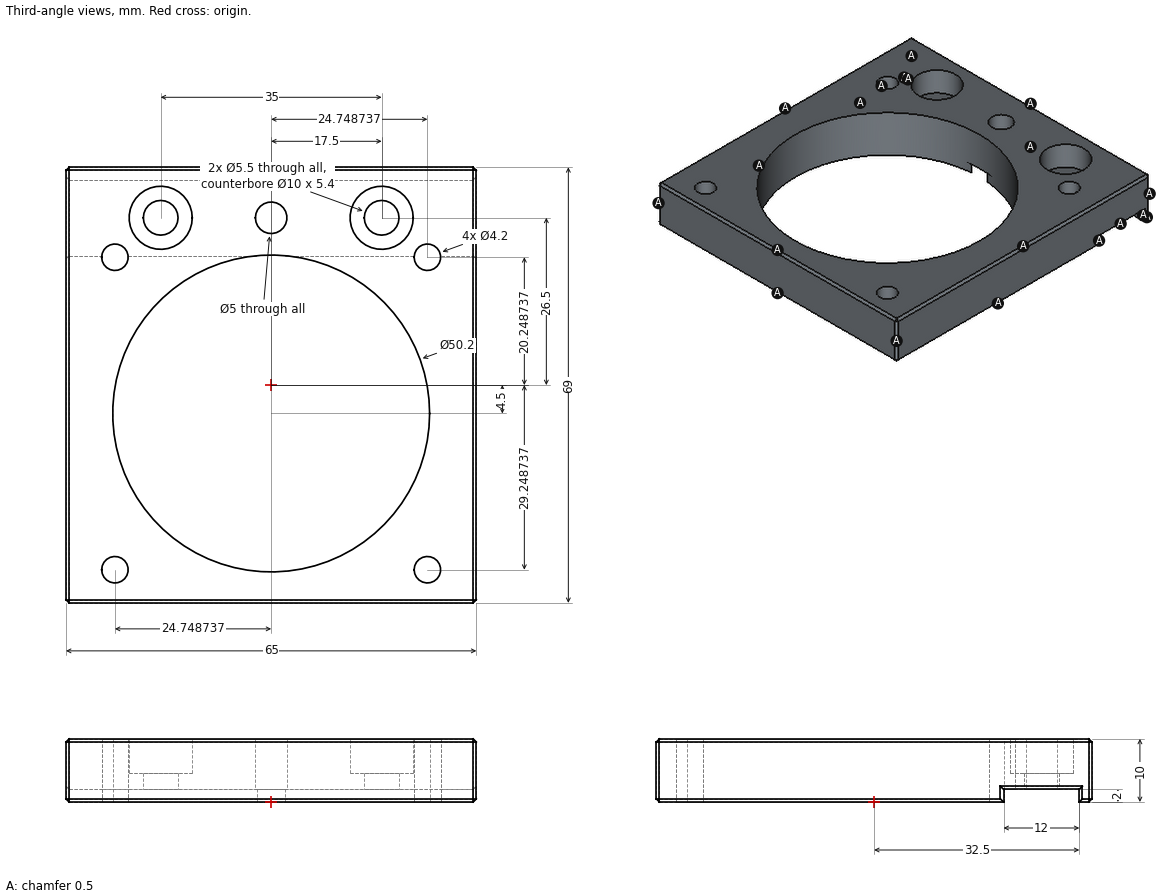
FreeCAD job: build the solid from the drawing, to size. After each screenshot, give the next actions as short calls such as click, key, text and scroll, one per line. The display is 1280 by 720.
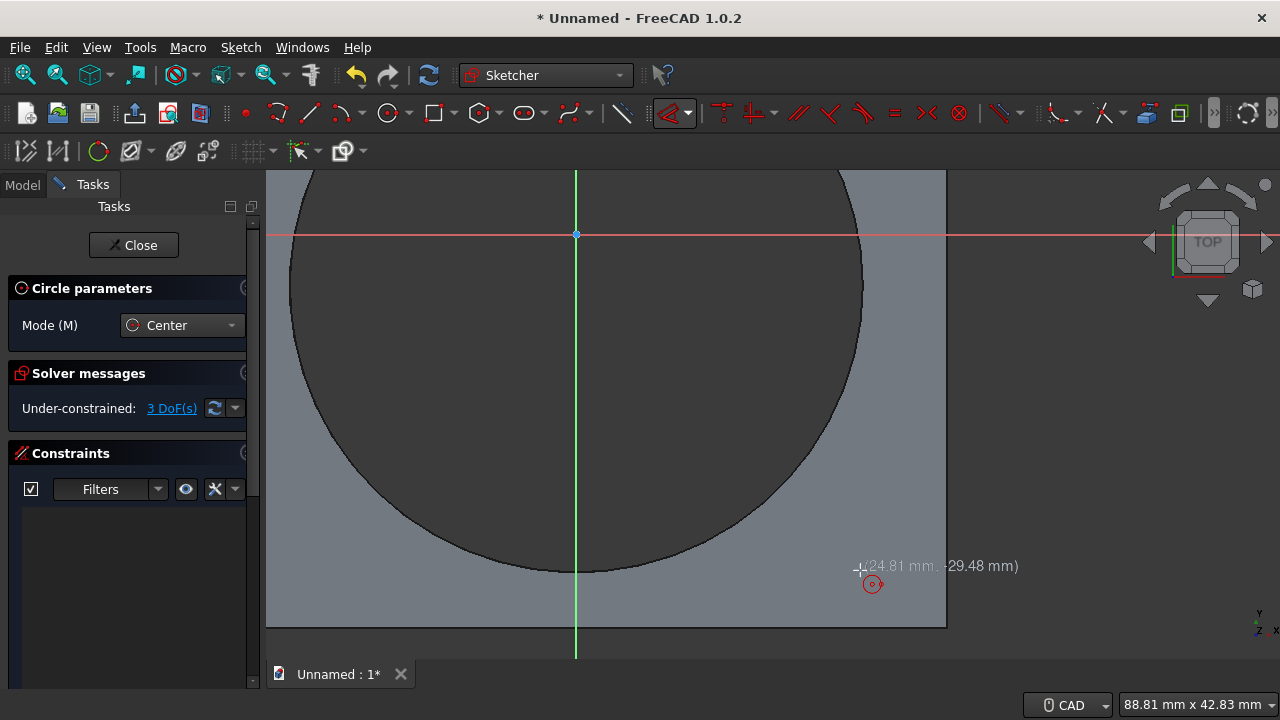
click(859, 568)
click(876, 552)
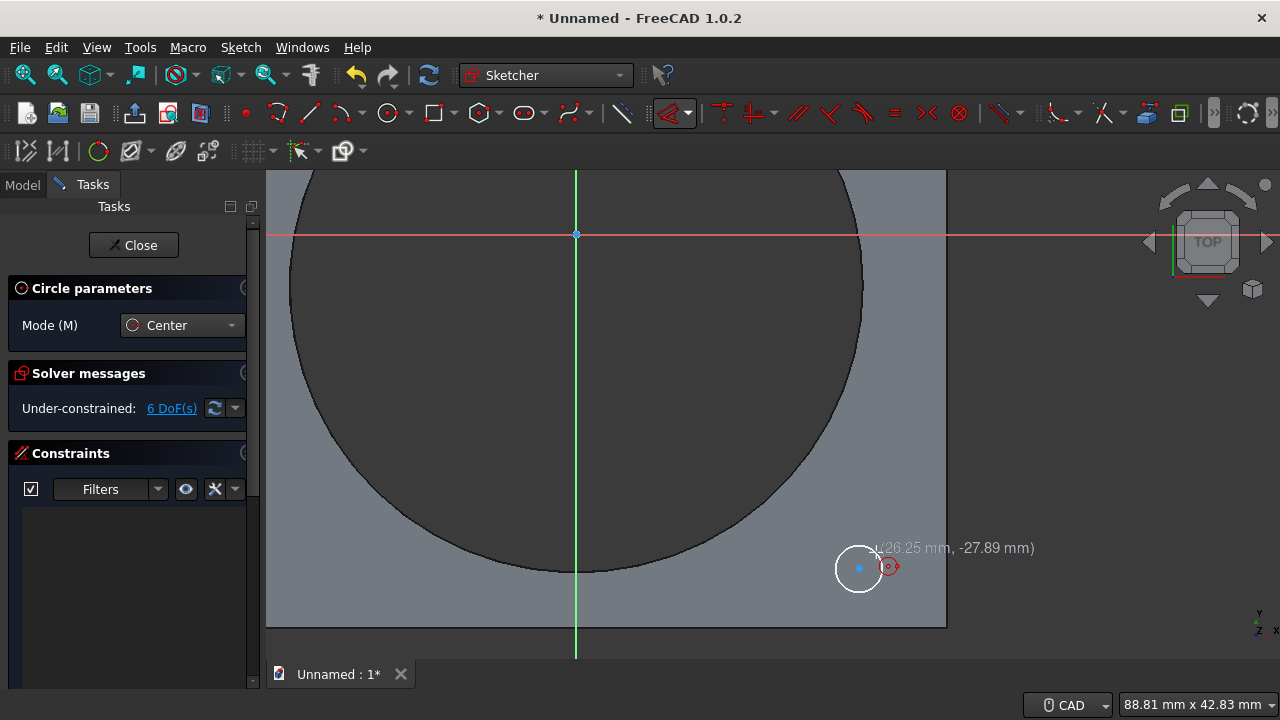
scroll(860, 571, down, 3)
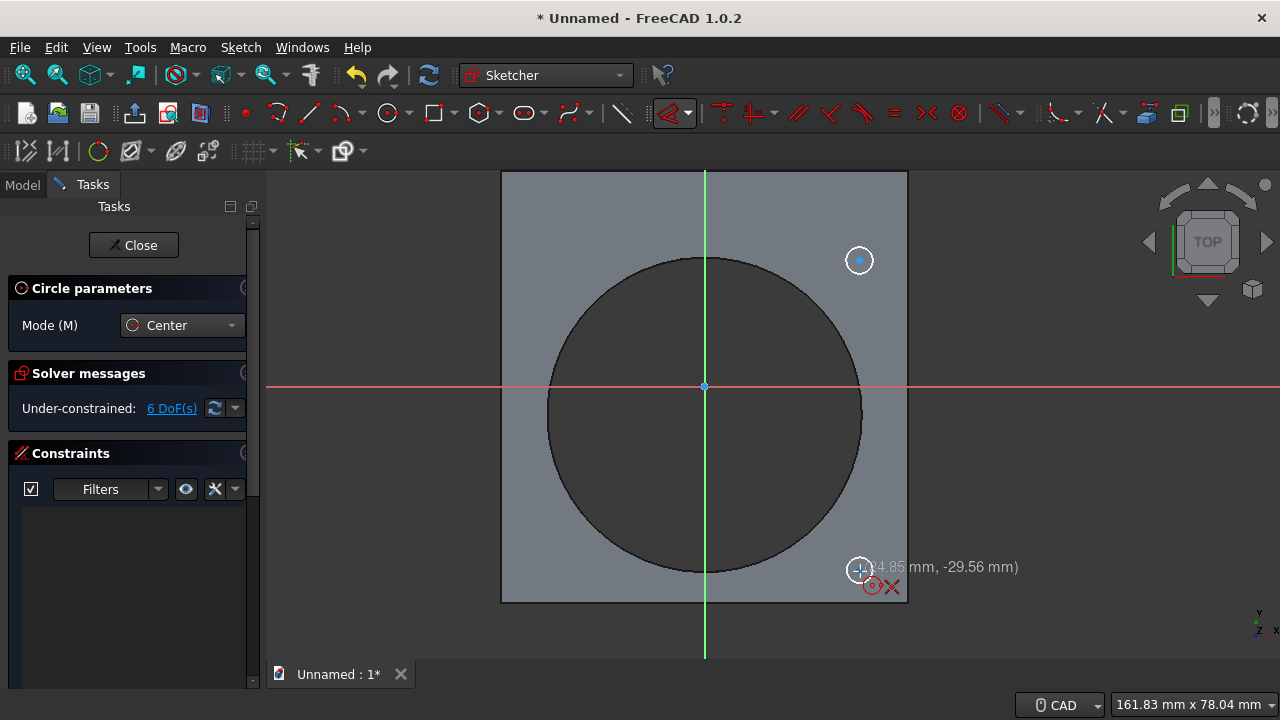
scroll(549, 570, up, 3)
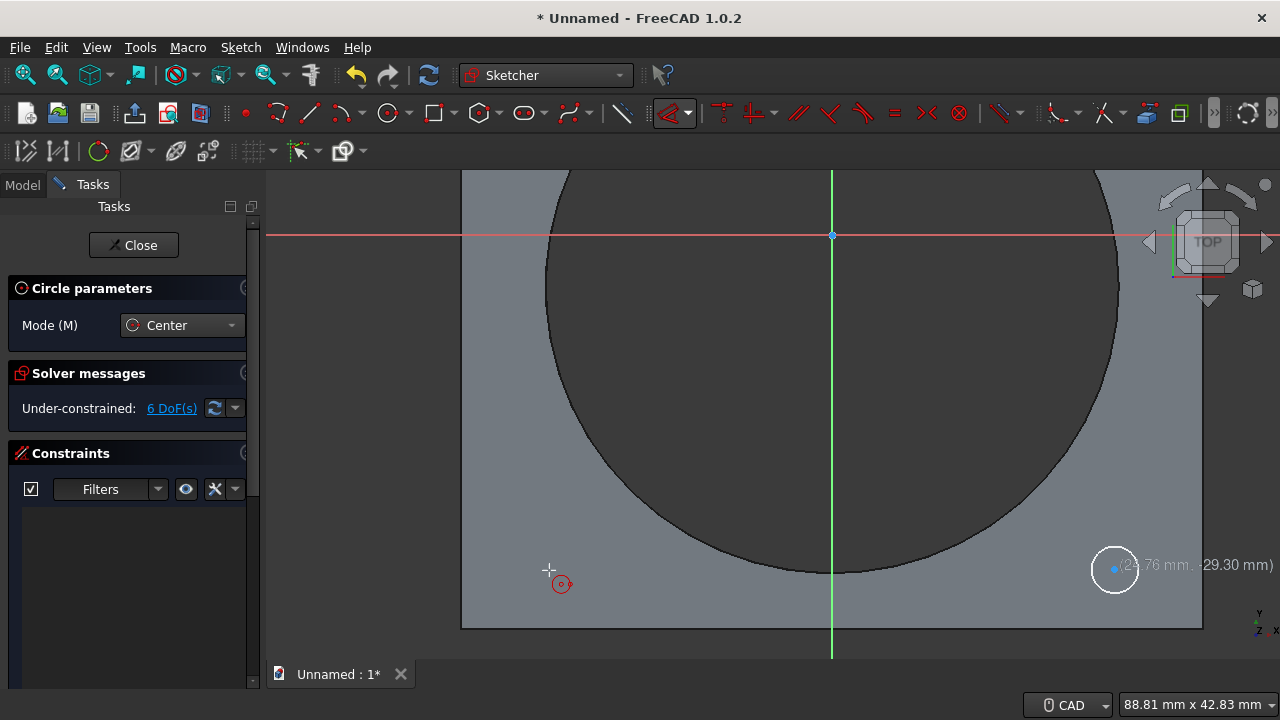
click(550, 569)
click(567, 552)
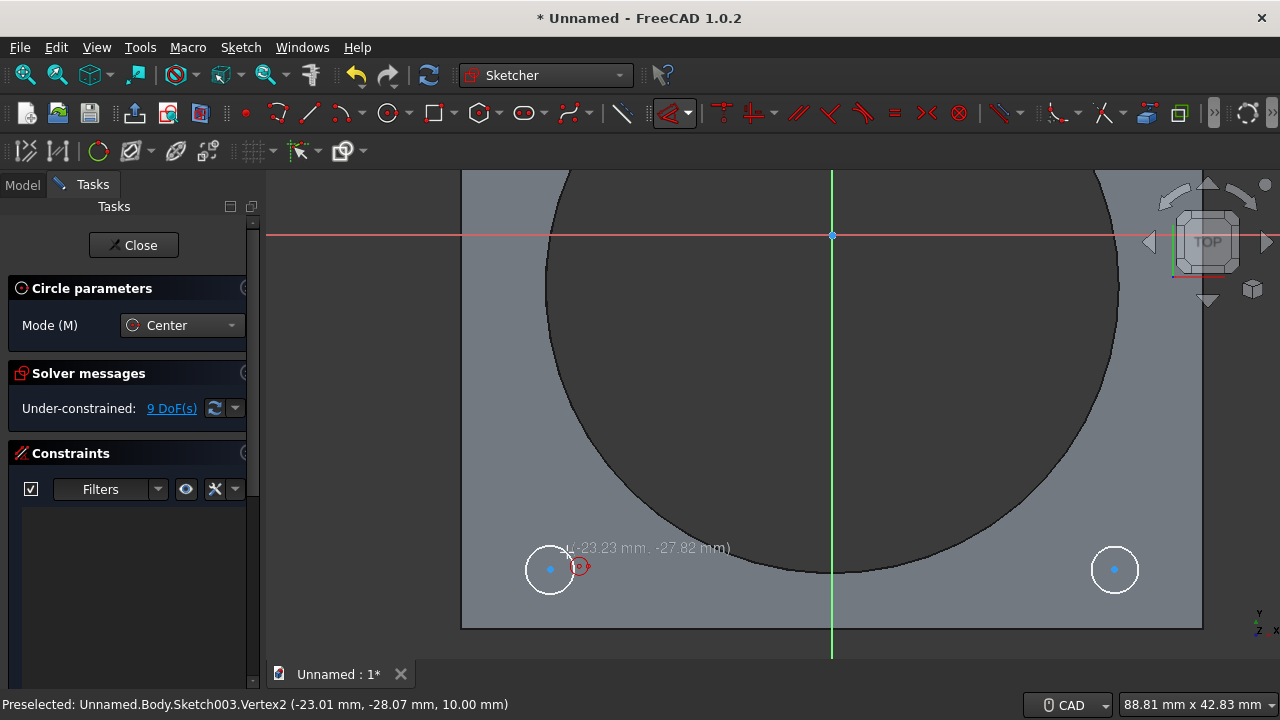
scroll(549, 570, down, 3)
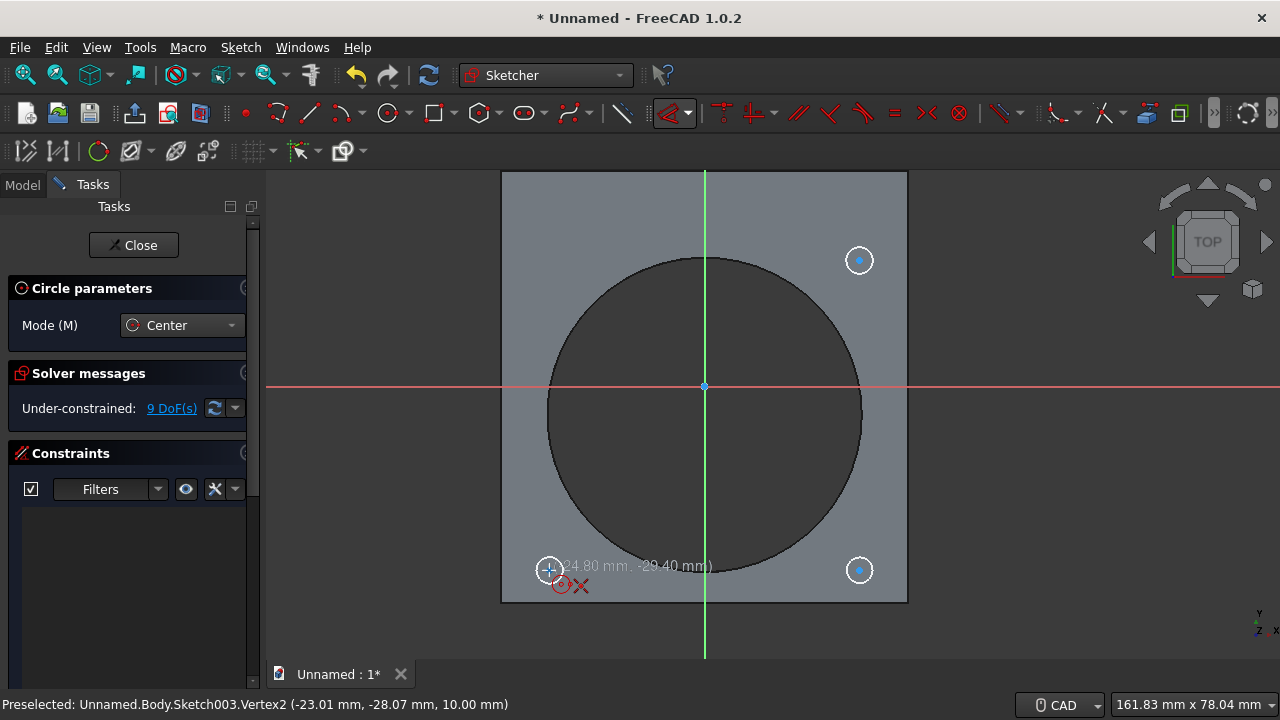
scroll(549, 260, up, 3)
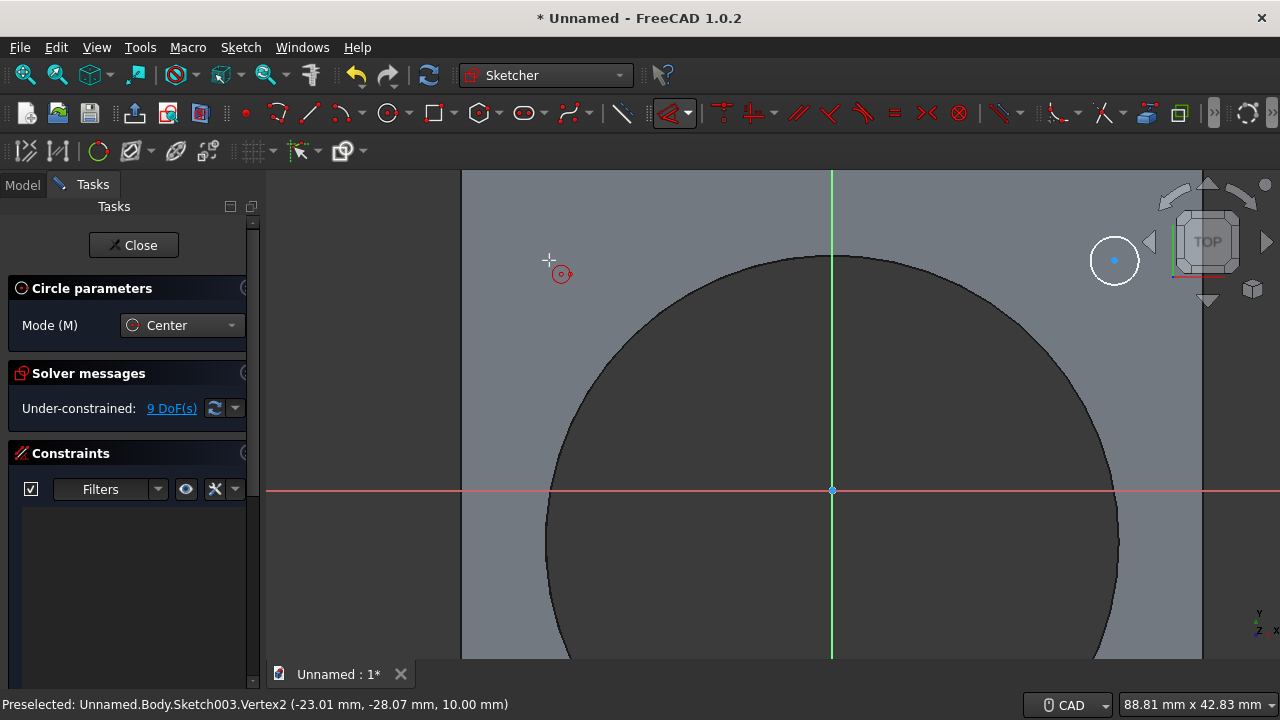
click(550, 260)
click(567, 243)
key(Escape)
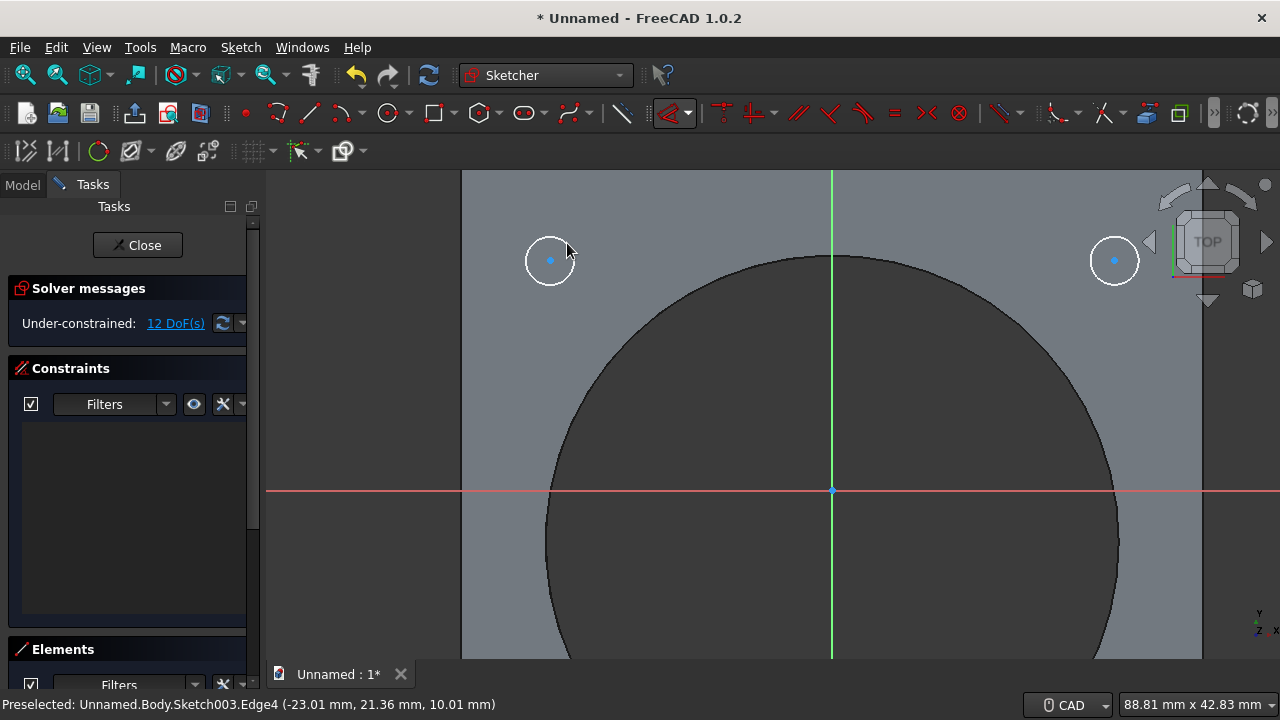
click(1098, 244)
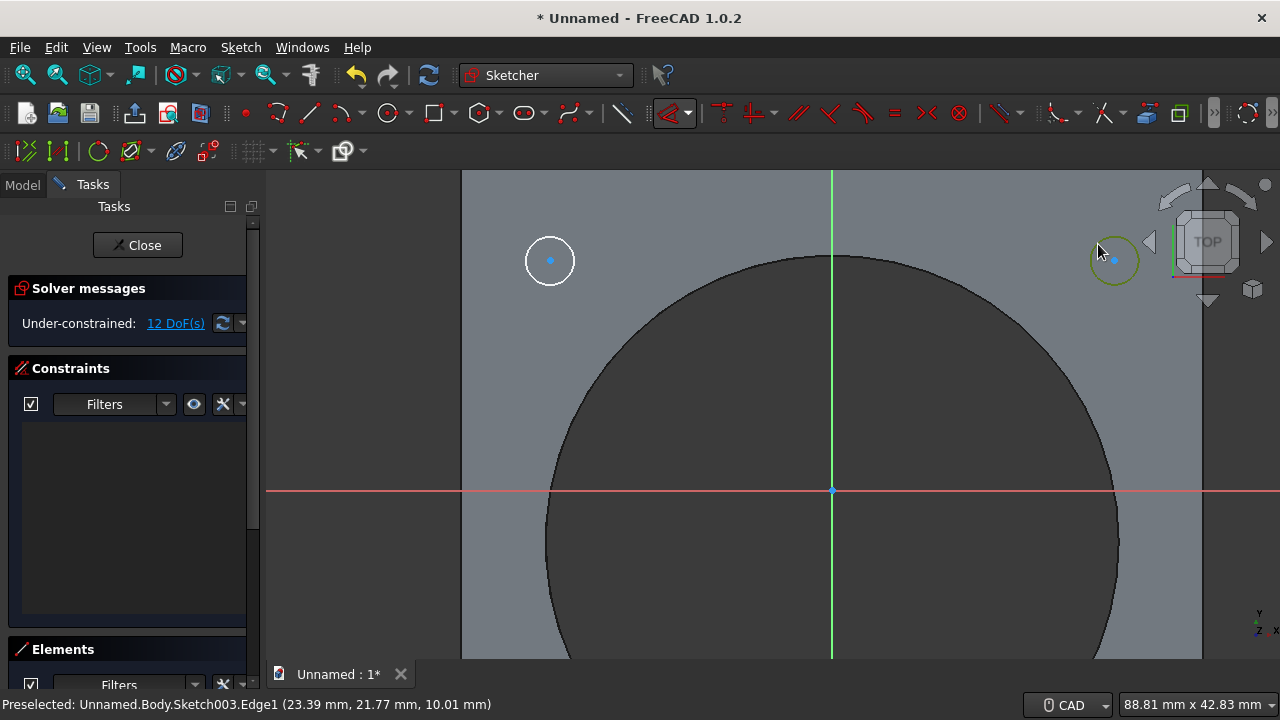
scroll(549, 259, down, 3)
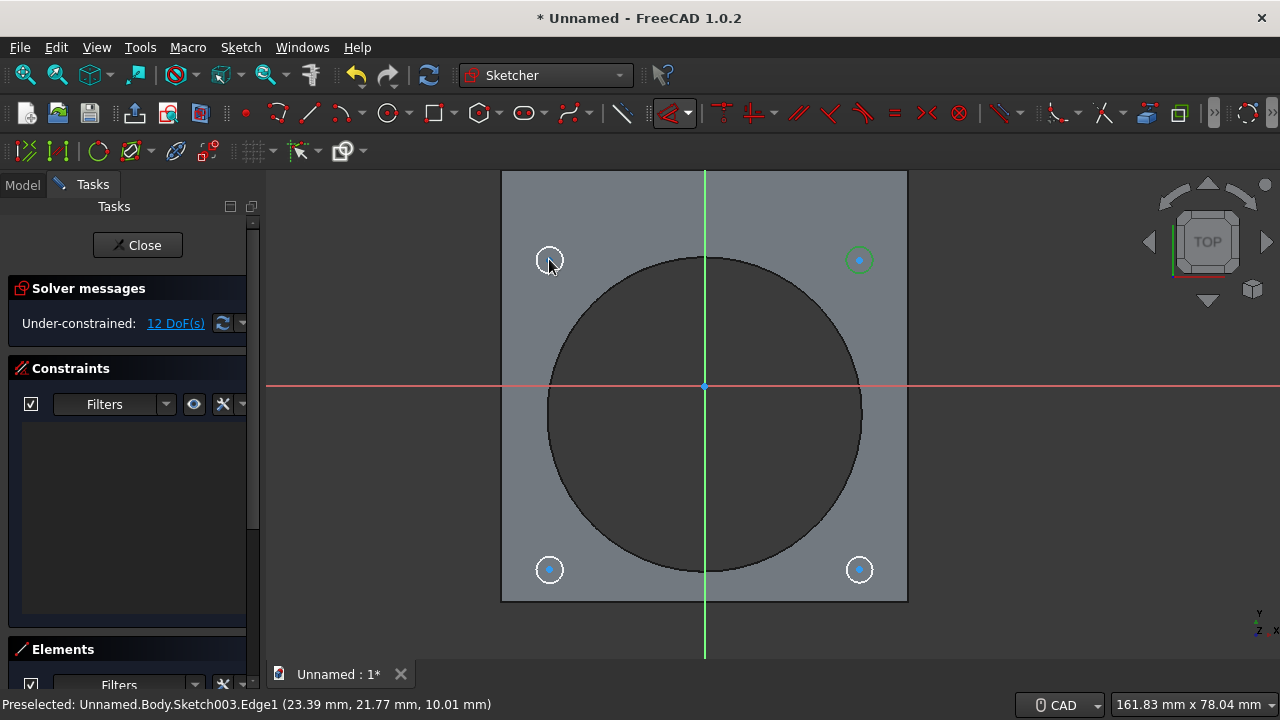
click(869, 561)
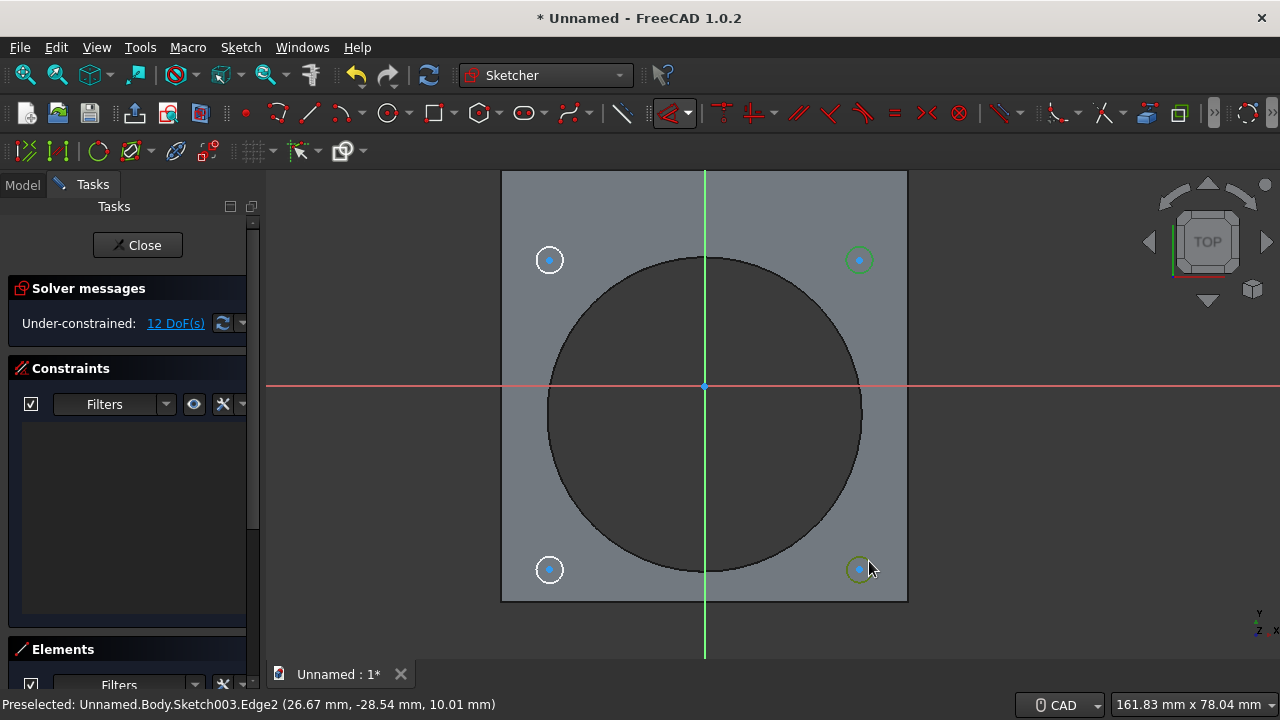
click(559, 561)